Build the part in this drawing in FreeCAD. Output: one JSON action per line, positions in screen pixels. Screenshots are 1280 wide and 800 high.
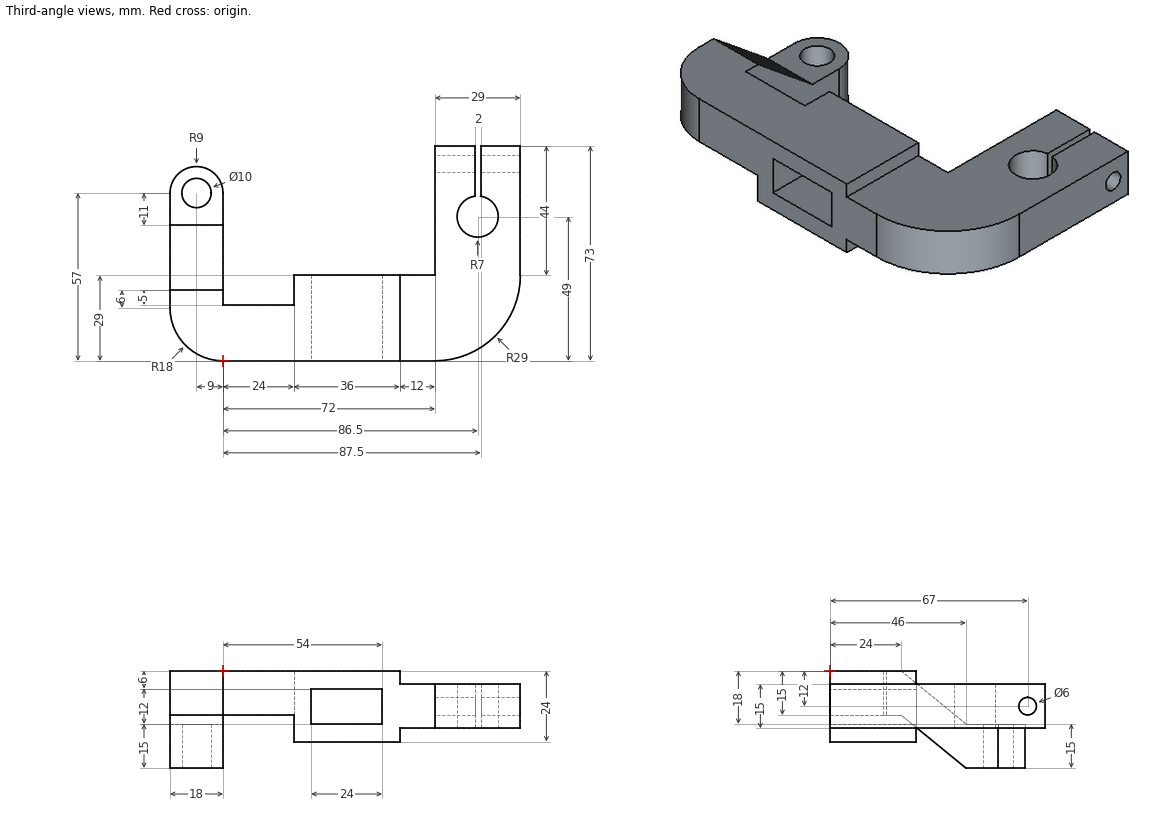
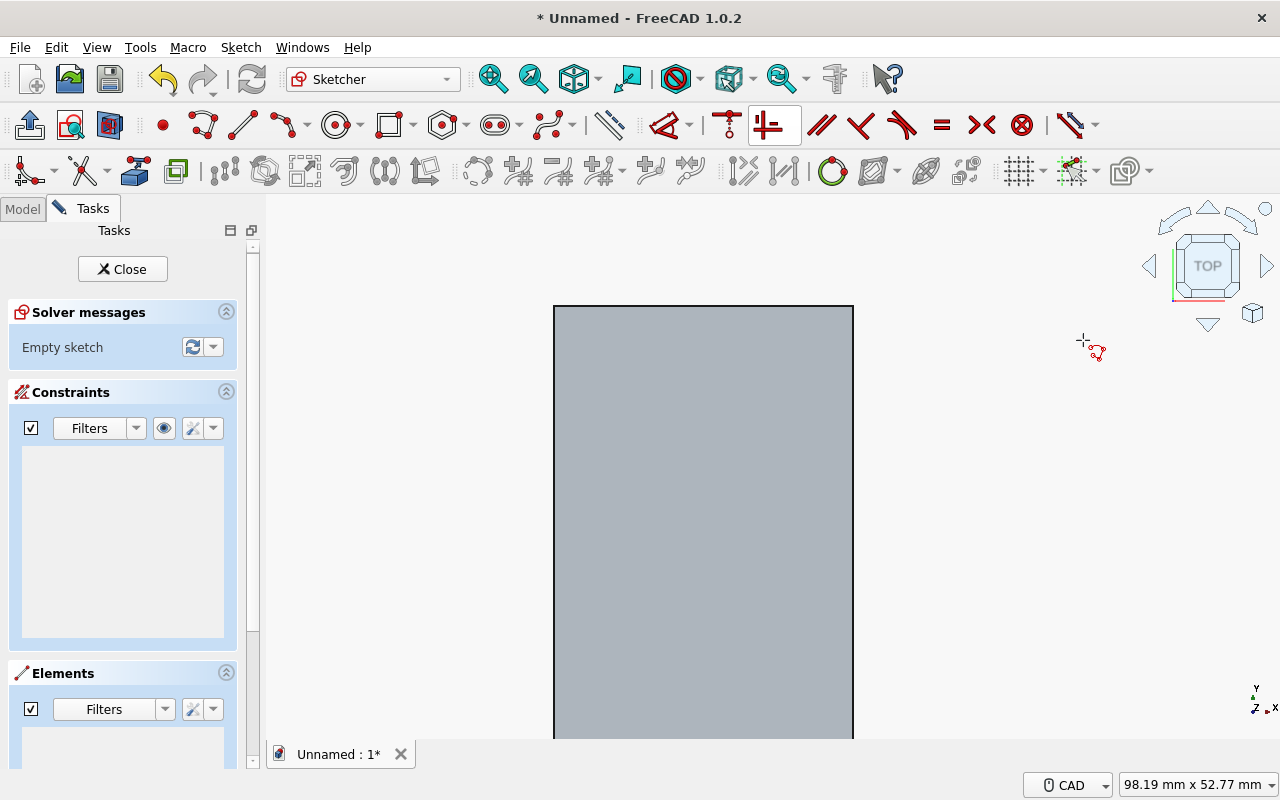
{"action": "left_click", "coordinate": [714, 483]}
{"action": "left_click", "coordinate": [714, 306]}
{"action": "left_click", "coordinate": [693, 306]}
{"action": "left_click", "coordinate": [693, 483]}
{"action": "right_click", "coordinate": [693, 483]}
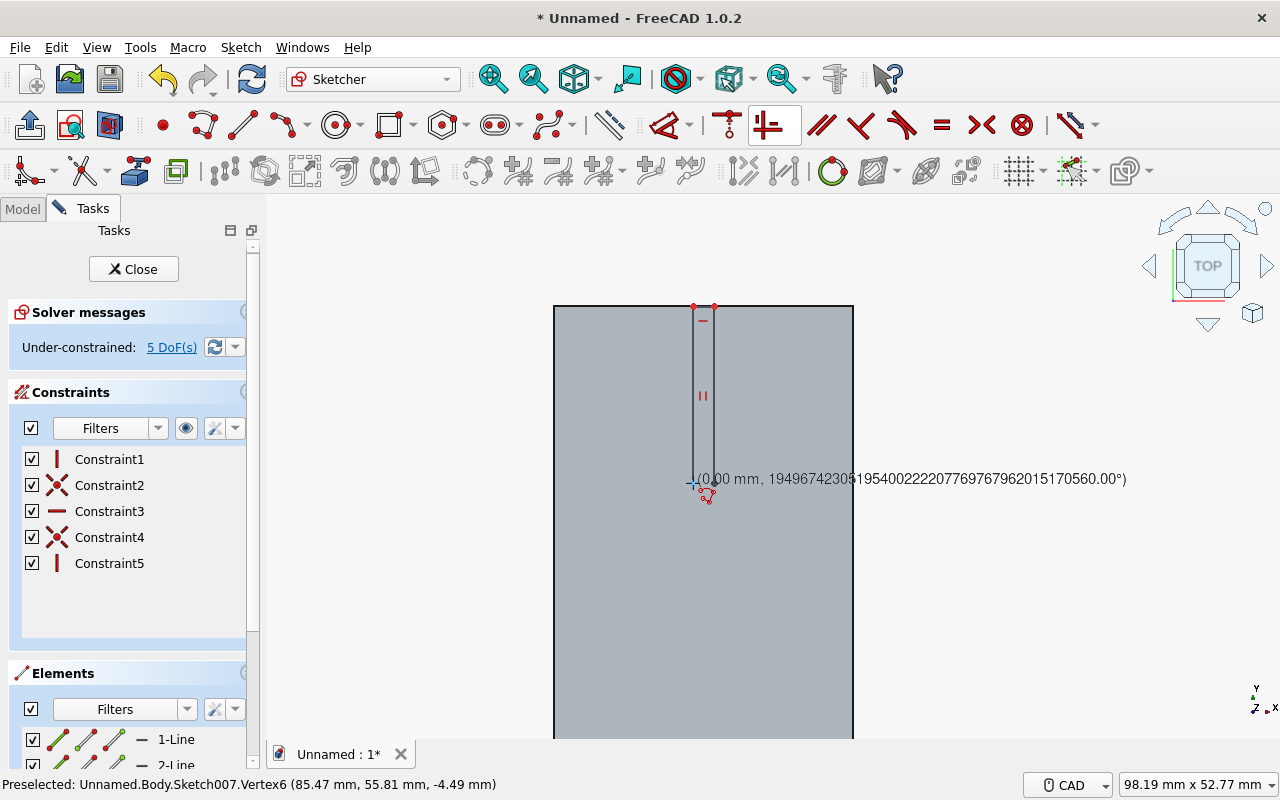
{"action": "key", "text": "g 3 a"}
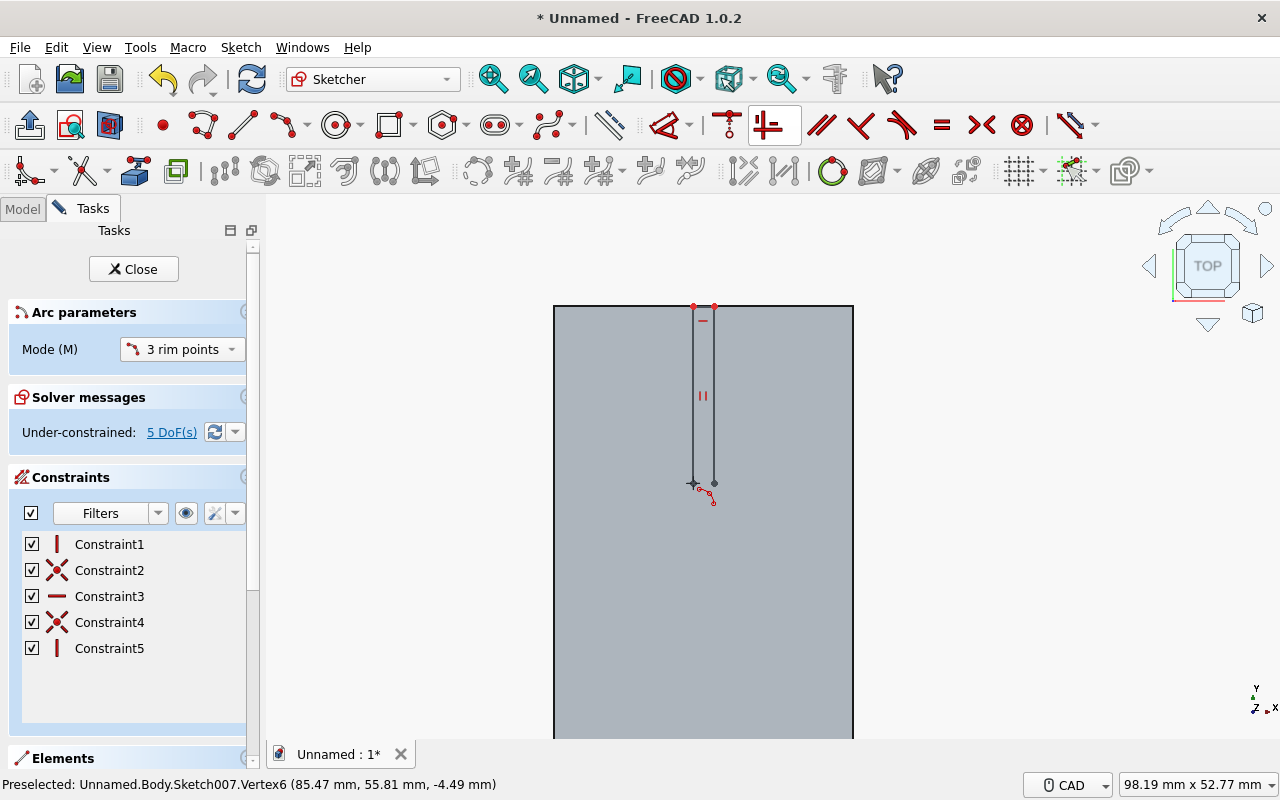
{"action": "left_click", "coordinate": [693, 484]}
{"action": "left_click", "coordinate": [714, 484]}
{"action": "left_click", "coordinate": [704, 627]}
{"action": "key", "text": "Escape"}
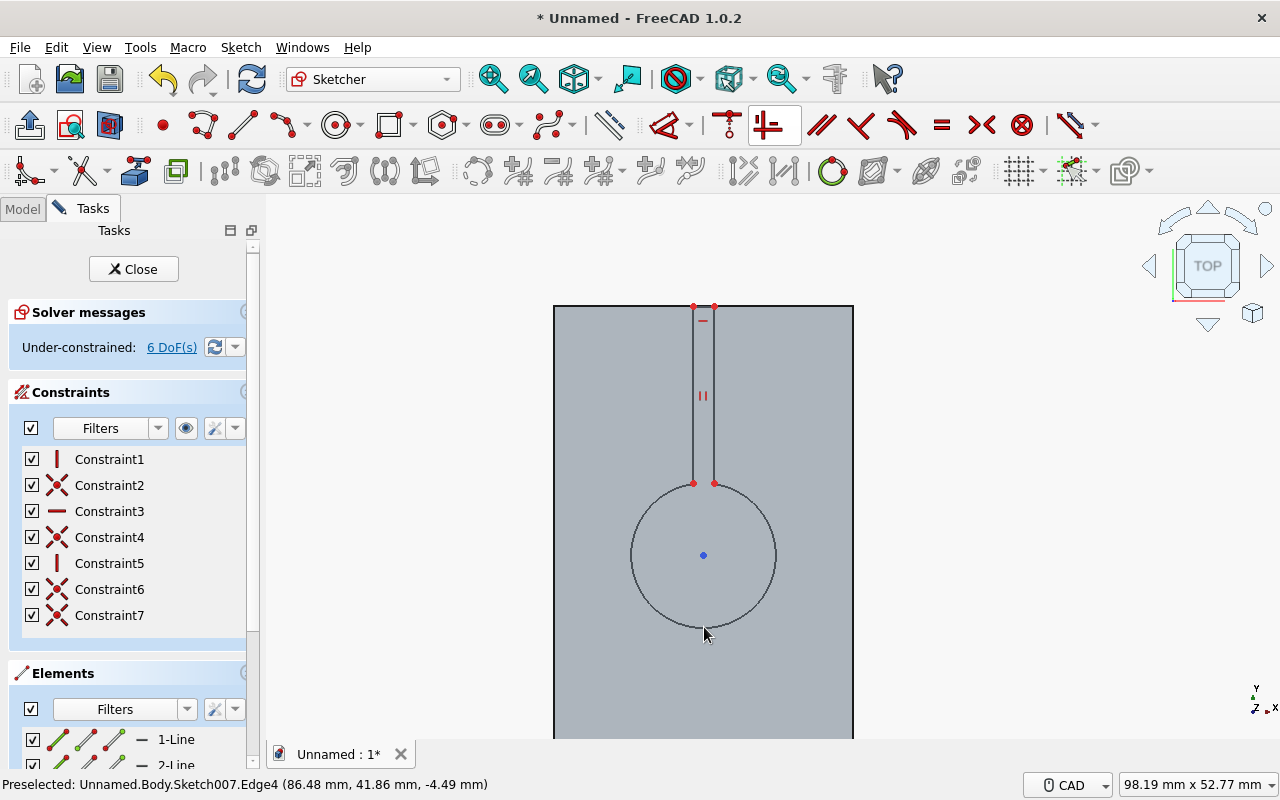
{"action": "left_click", "coordinate": [664, 126]}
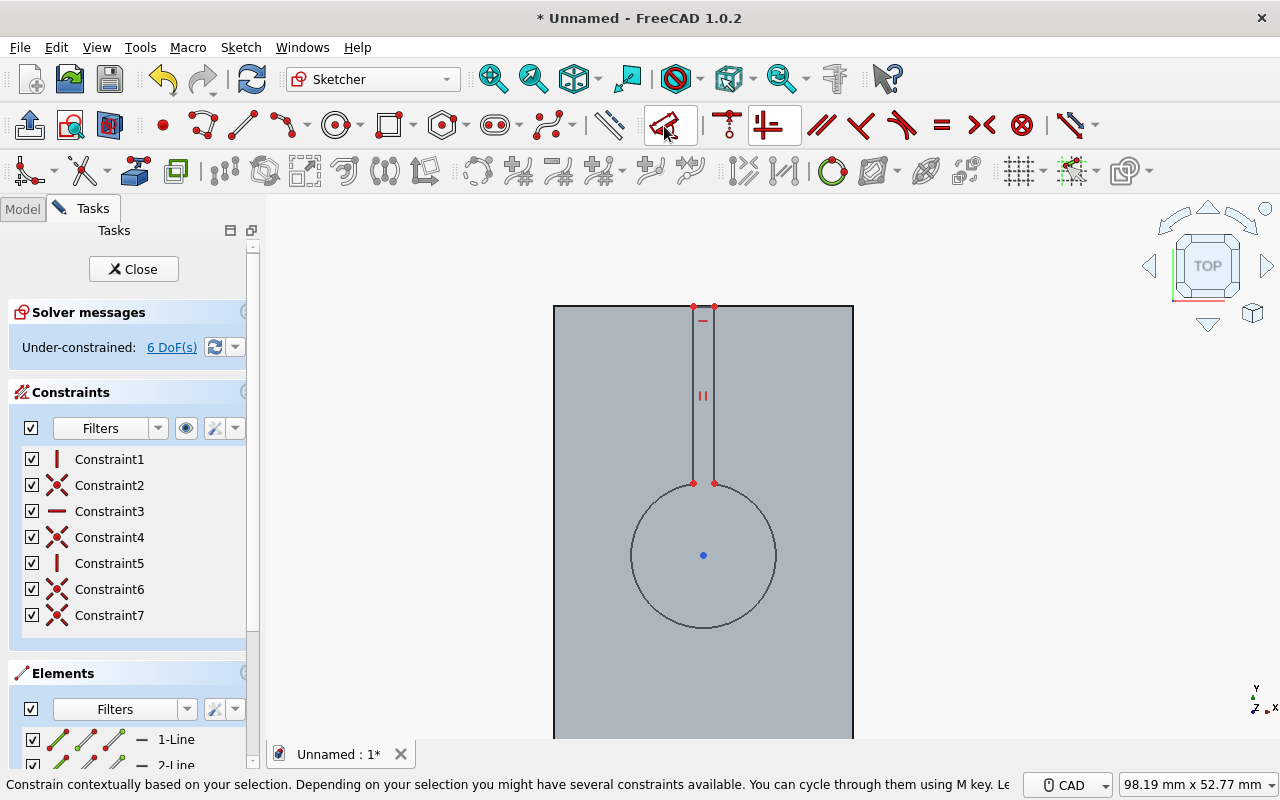
{"action": "left_click", "coordinate": [636, 582]}
{"action": "left_click", "coordinate": [606, 594]}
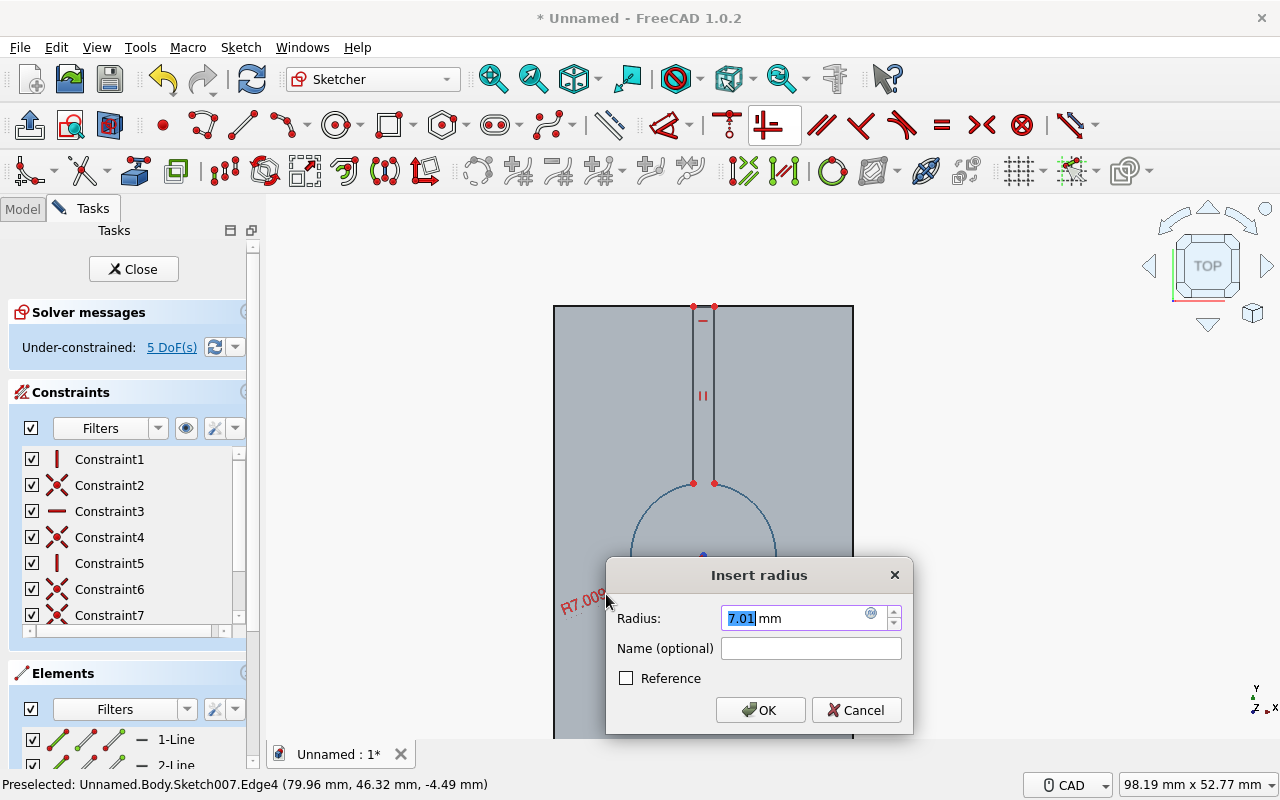
{"action": "type", "text": "7"}
{"action": "key", "text": "Return"}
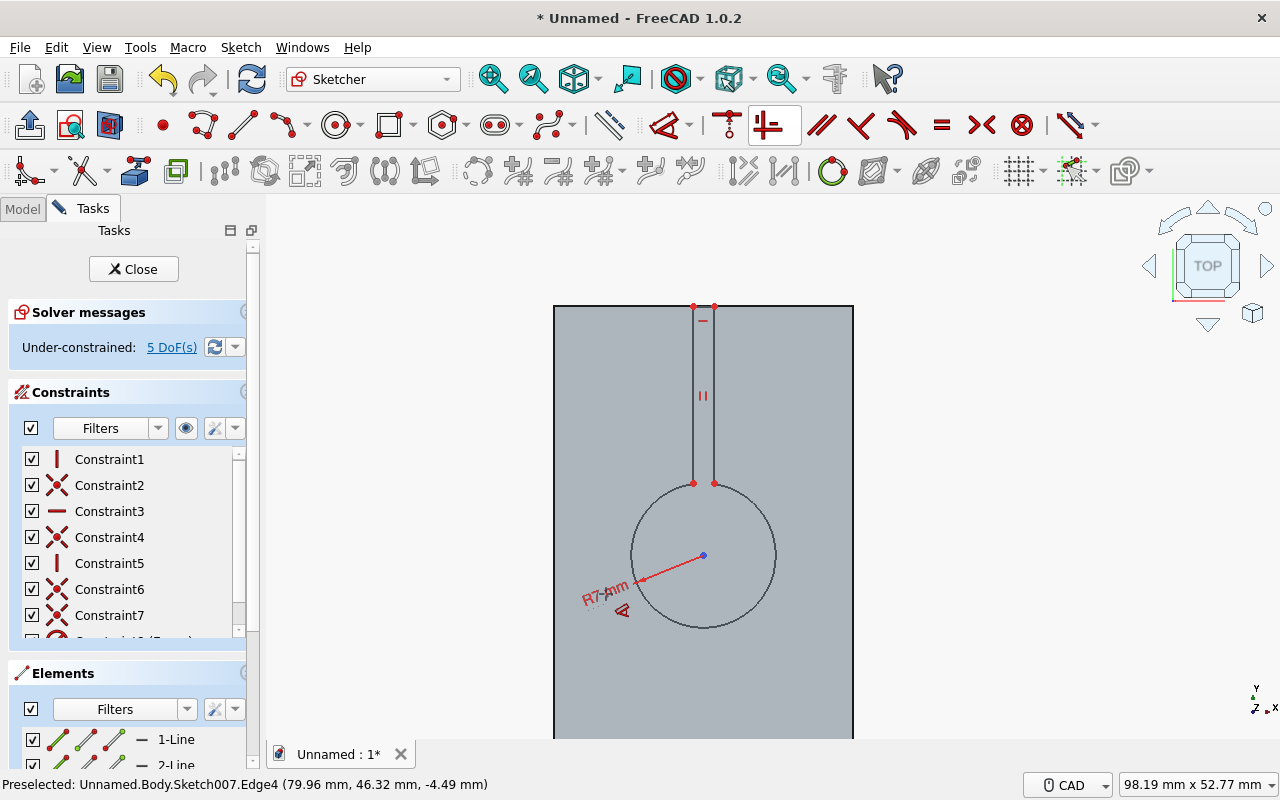
{"action": "scroll", "coordinate": [704, 307], "scroll_direction": "up", "scroll_amount": 4}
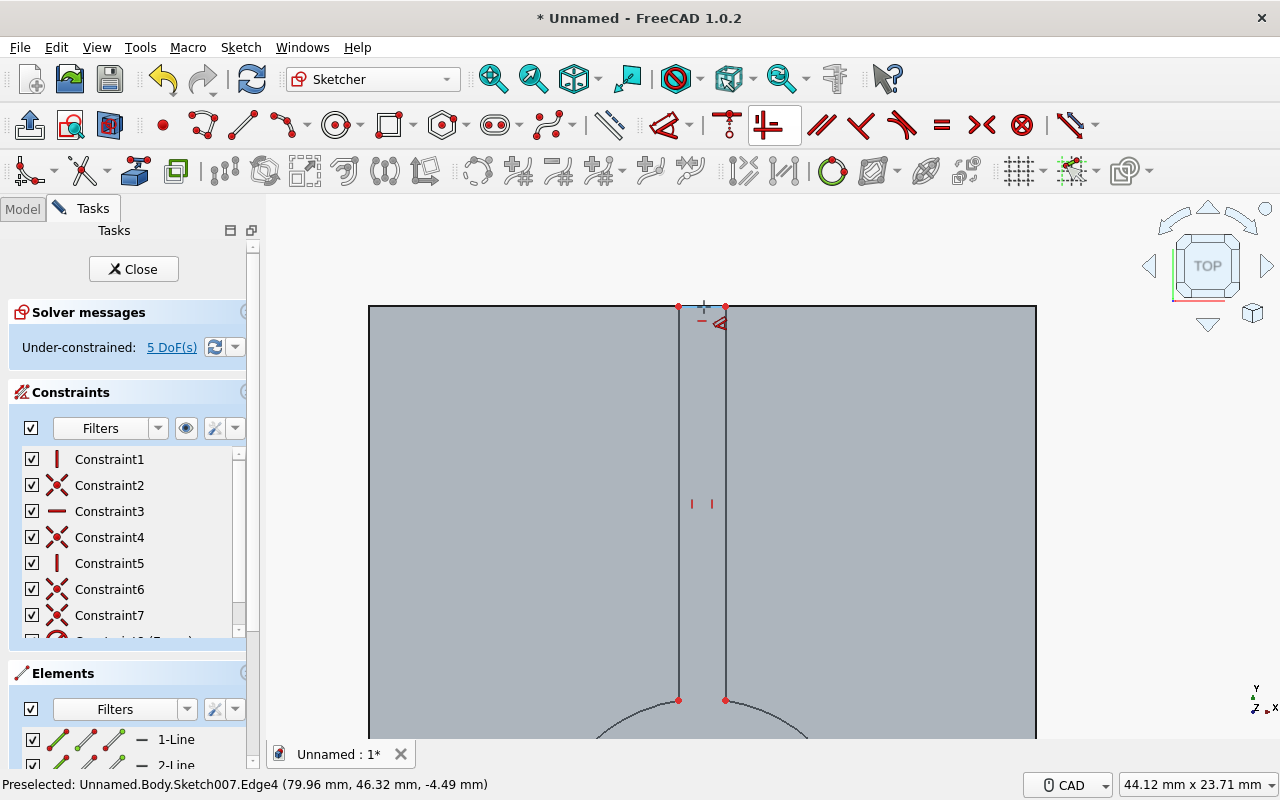
{"action": "left_click", "coordinate": [702, 307]}
{"action": "left_click", "coordinate": [702, 273]}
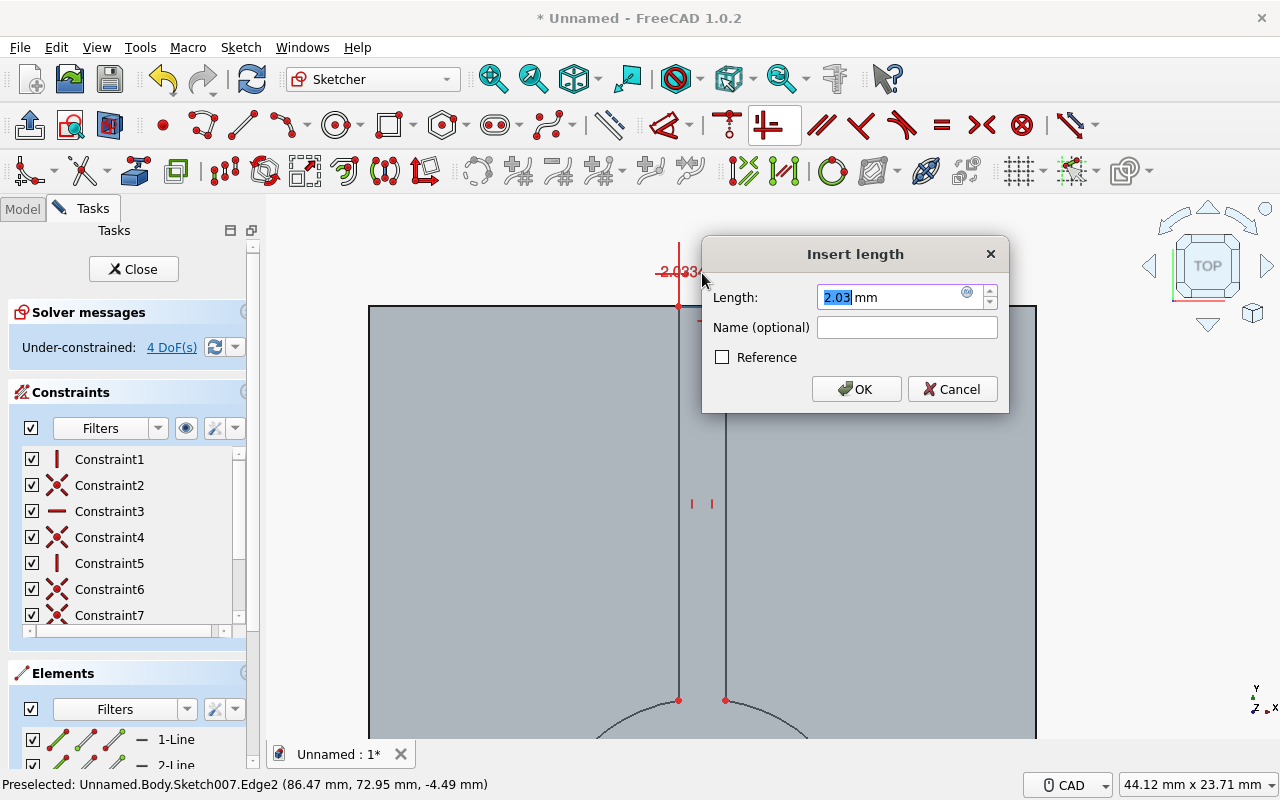
{"action": "type", "text": "2"}
{"action": "key", "text": "Return"}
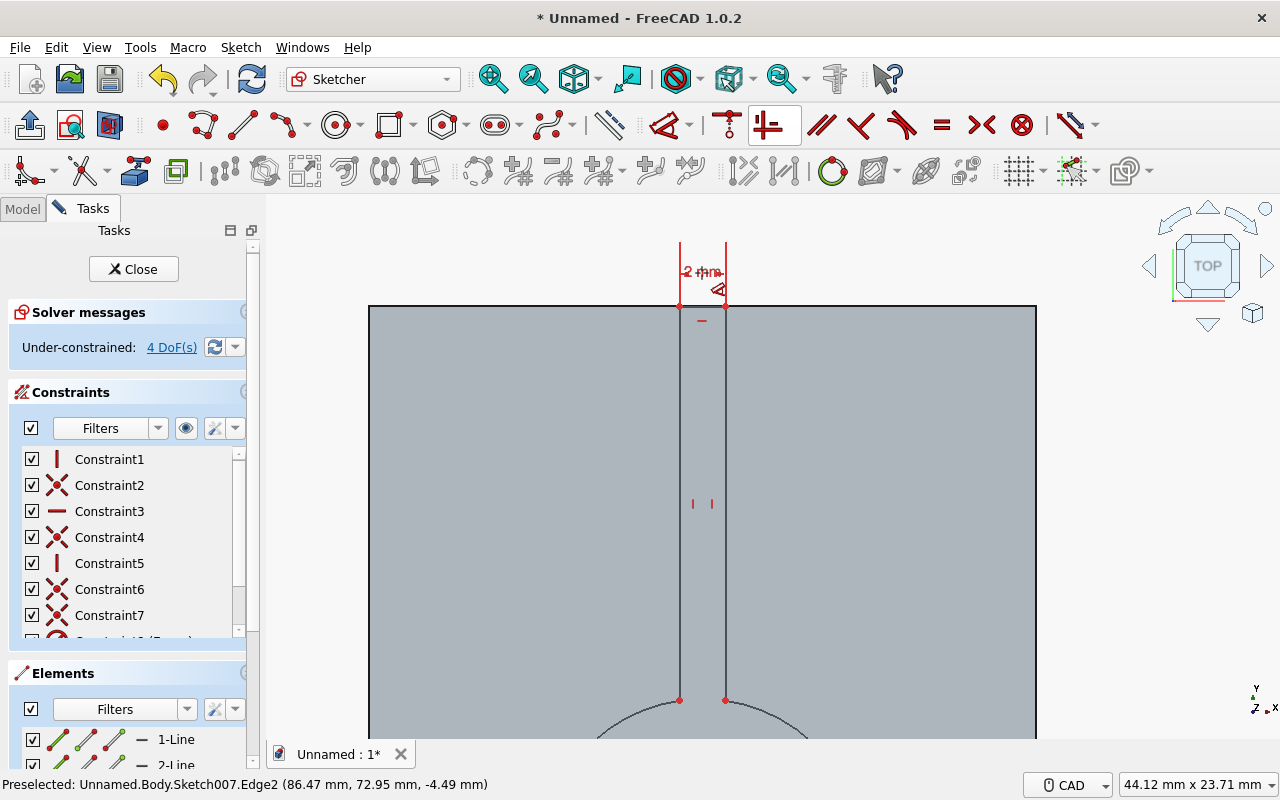
{"action": "left_click", "coordinate": [726, 307]}
{"action": "left_click", "coordinate": [760, 509]}